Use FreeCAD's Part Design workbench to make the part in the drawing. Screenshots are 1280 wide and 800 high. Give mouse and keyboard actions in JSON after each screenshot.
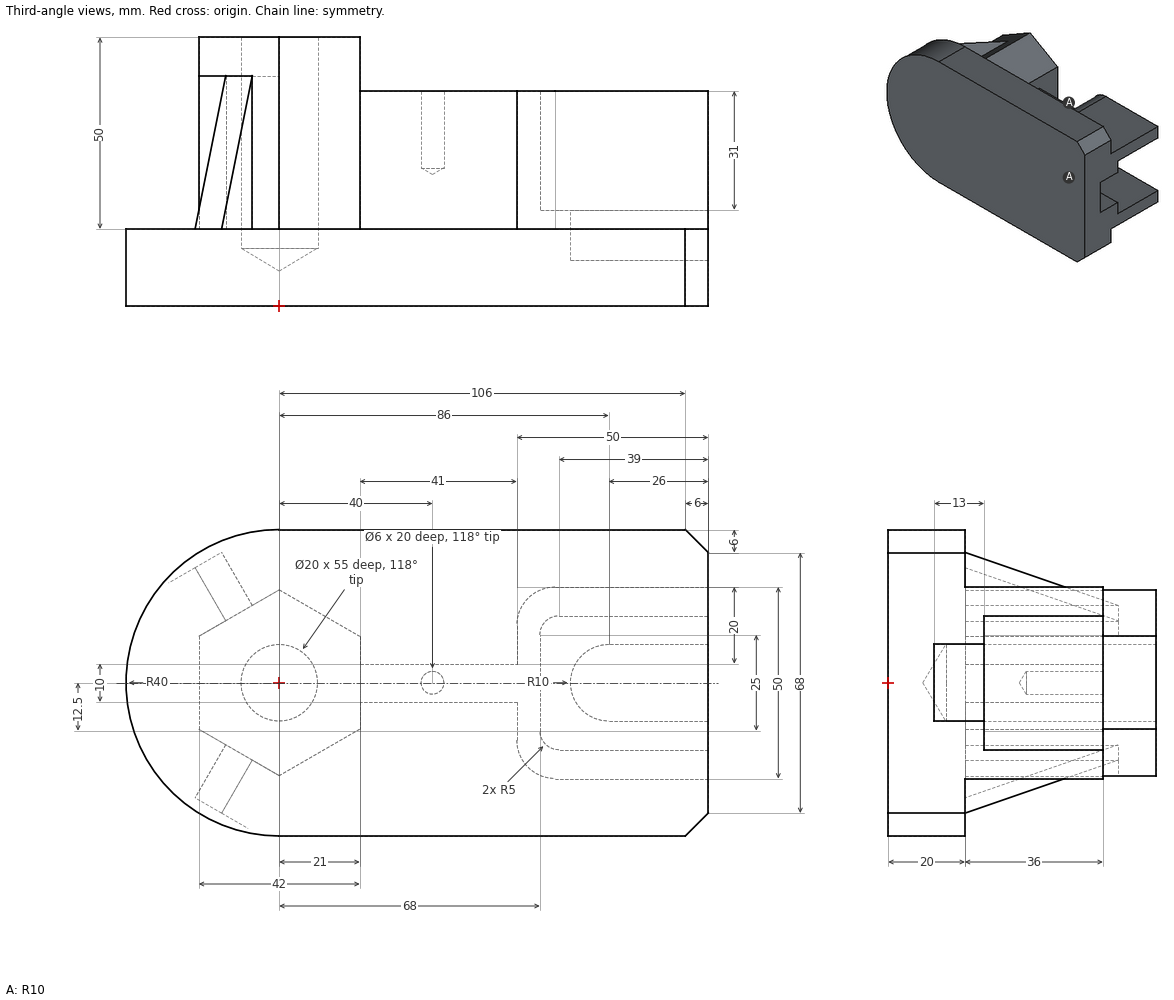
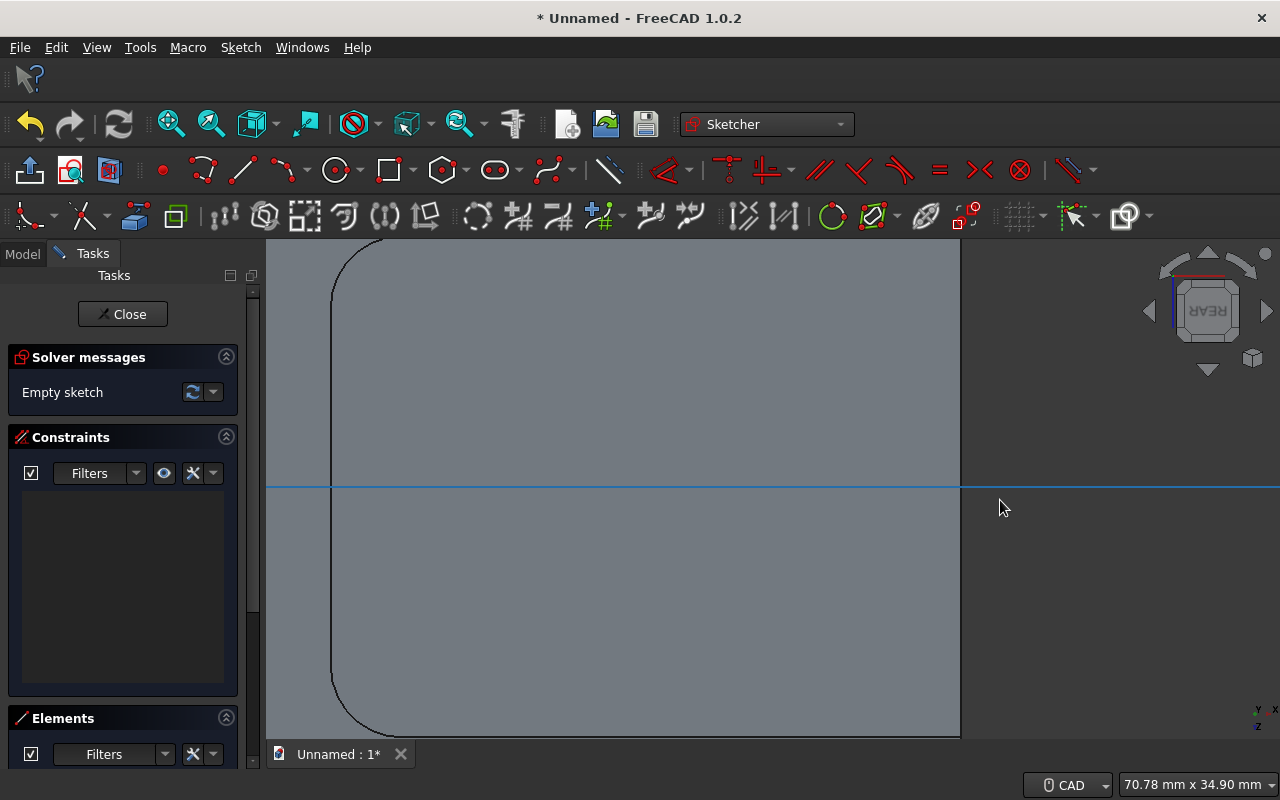
{"action": "left_click", "coordinate": [204, 170]}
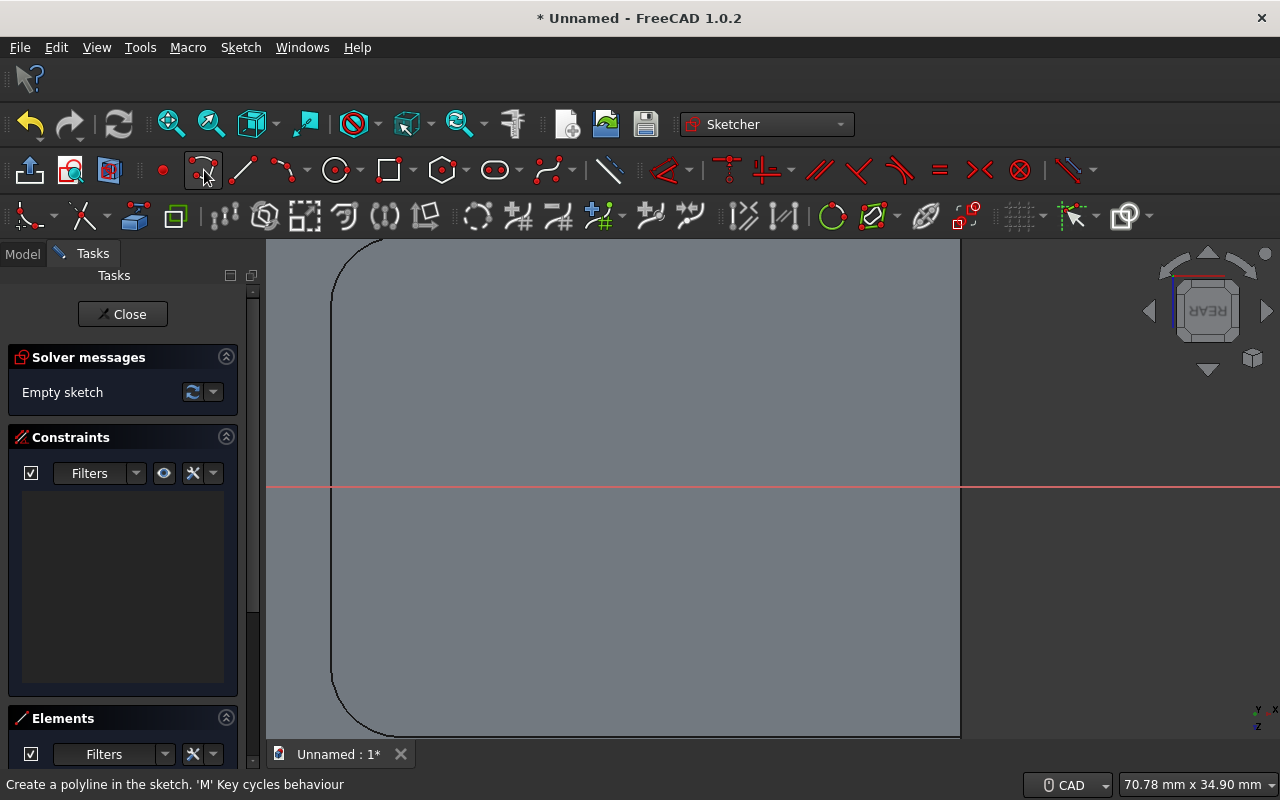
{"action": "left_click", "coordinate": [589, 630]}
{"action": "left_click", "coordinate": [961, 630]}
{"action": "left_click", "coordinate": [961, 344]}
{"action": "left_click", "coordinate": [589, 344]}
{"action": "right_click", "coordinate": [589, 344]}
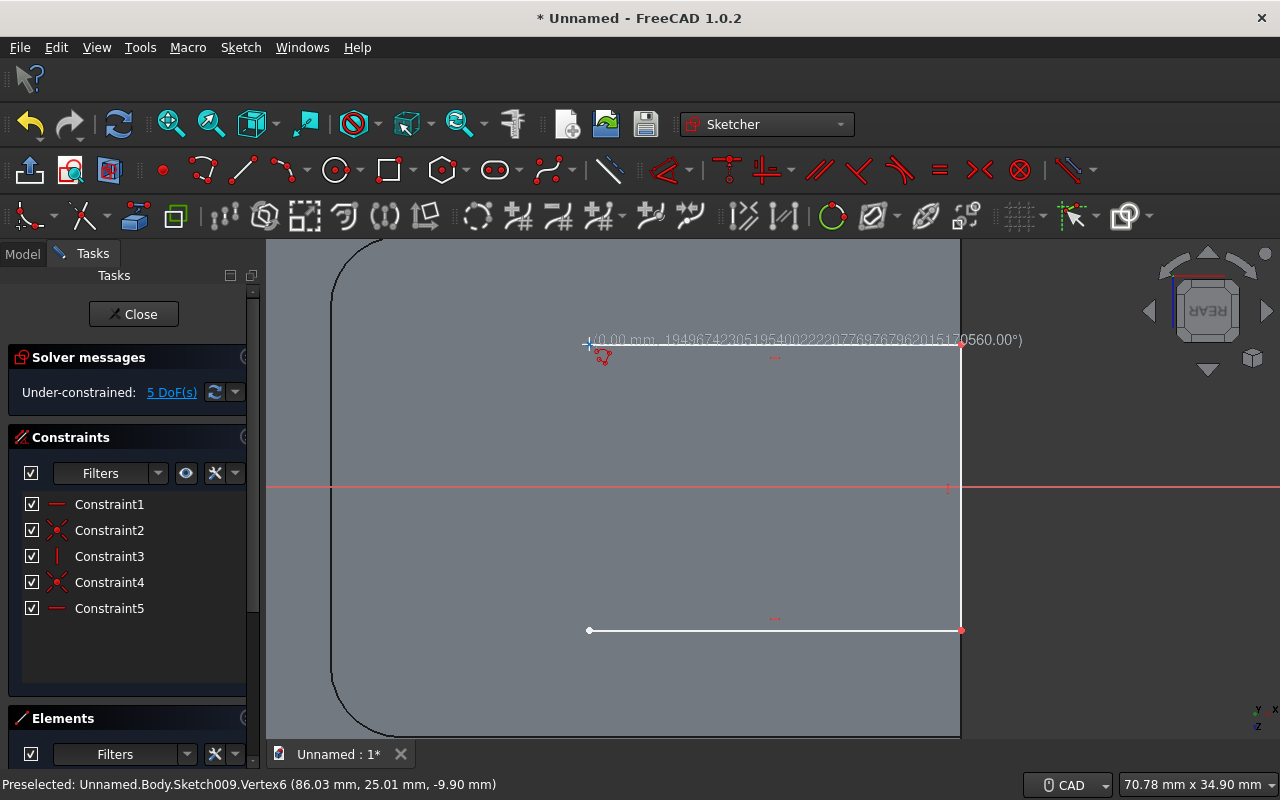
{"action": "left_click", "coordinate": [284, 170]}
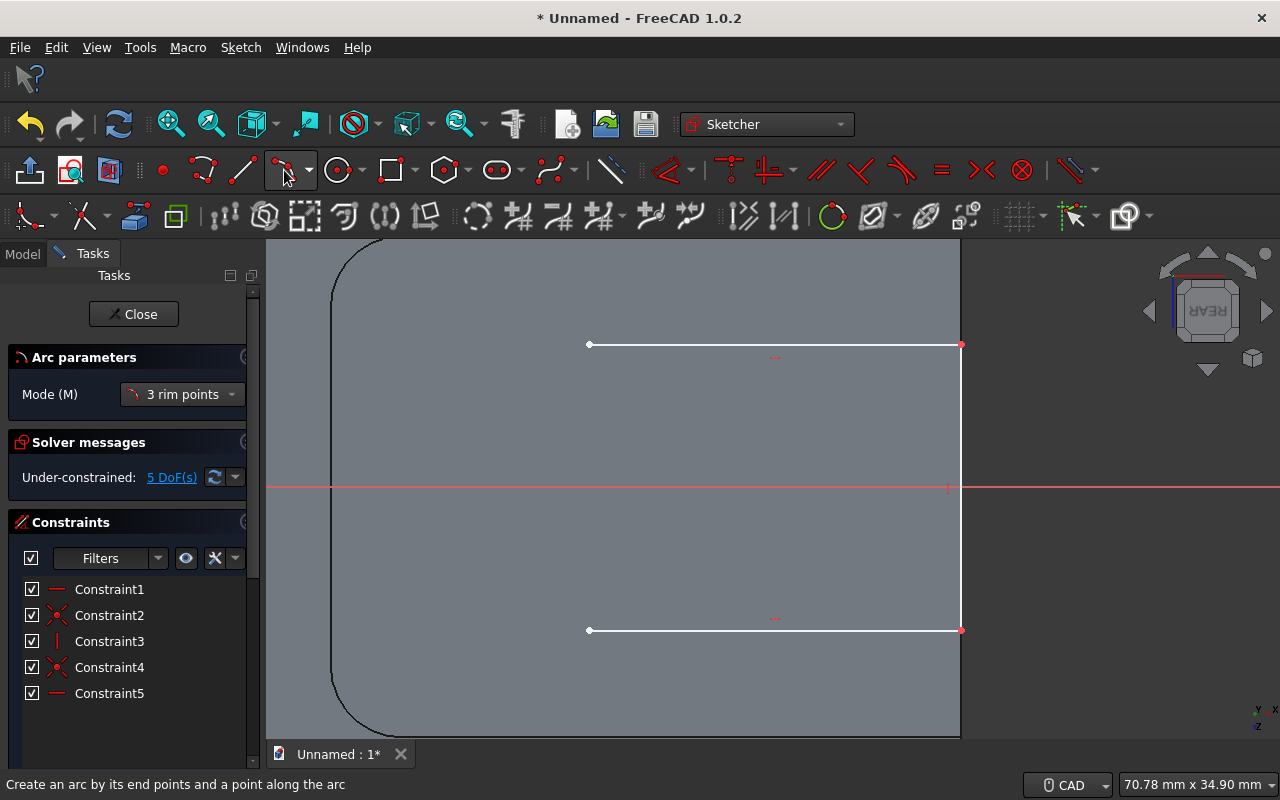
{"action": "left_click", "coordinate": [589, 345]}
{"action": "left_click", "coordinate": [589, 631]}
{"action": "left_click", "coordinate": [452, 442]}
{"action": "key", "text": "Escape"}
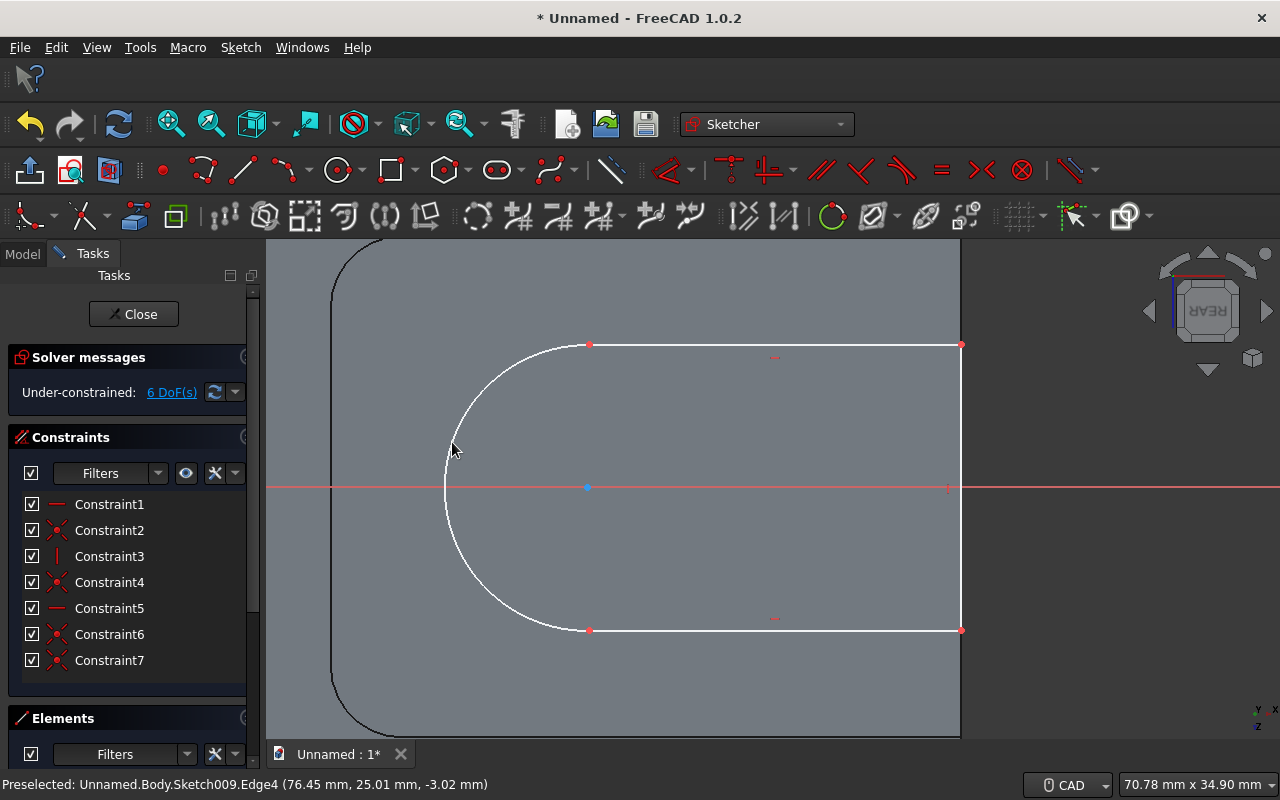
{"action": "left_click", "coordinate": [701, 631]}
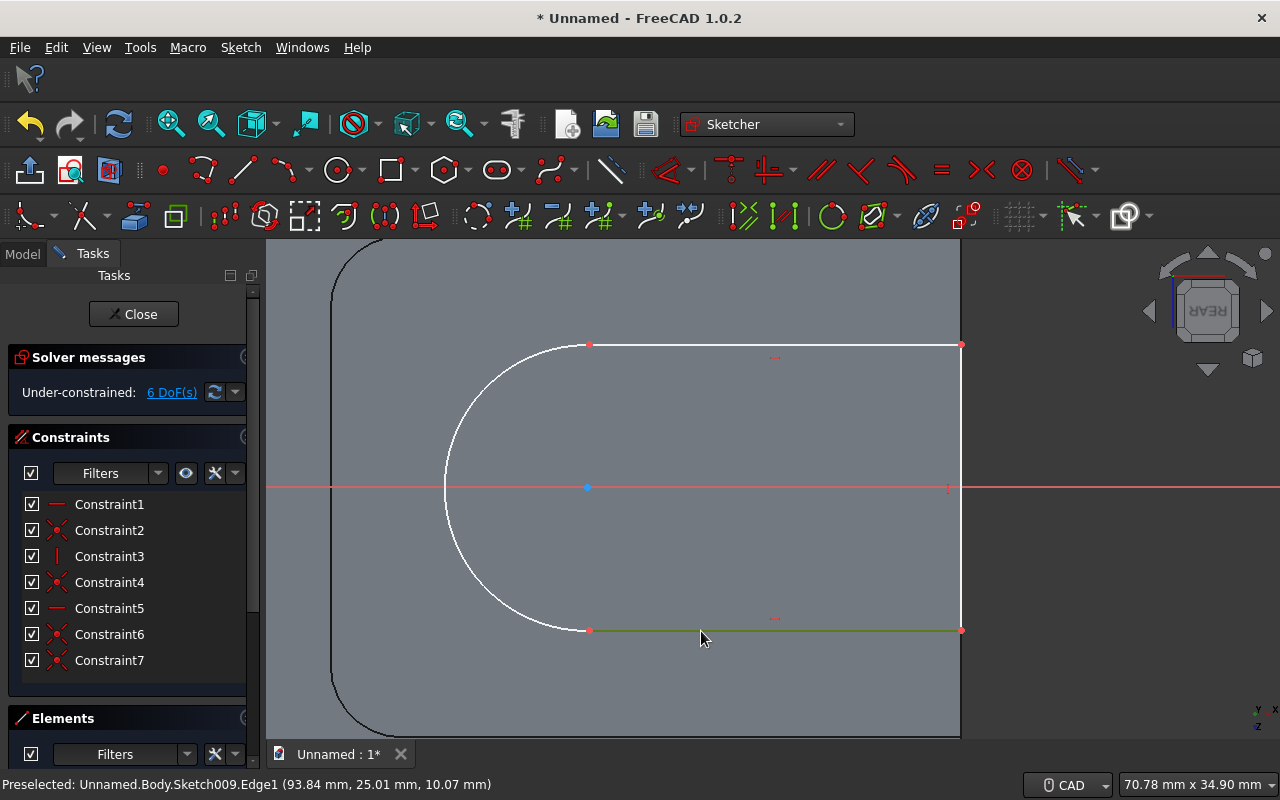
{"action": "left_click", "coordinate": [472, 404]}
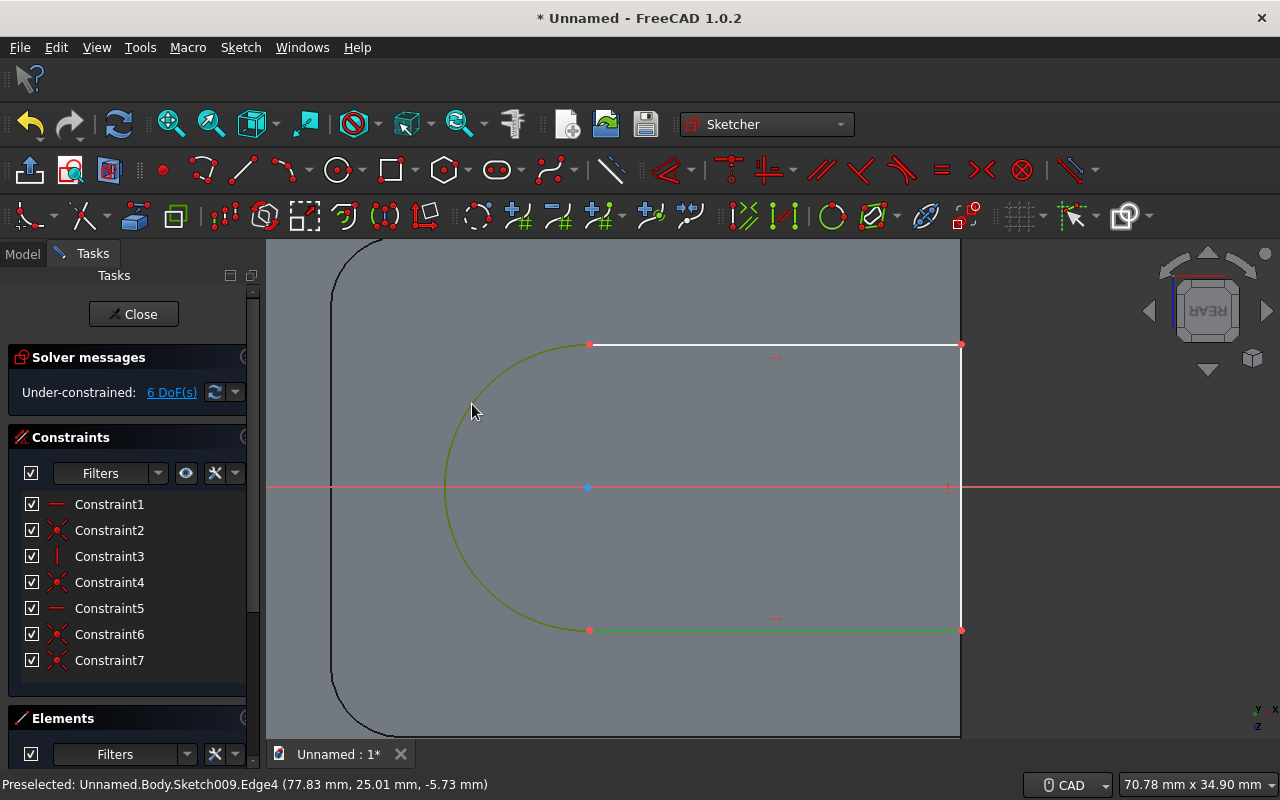
{"action": "left_click", "coordinate": [902, 170]}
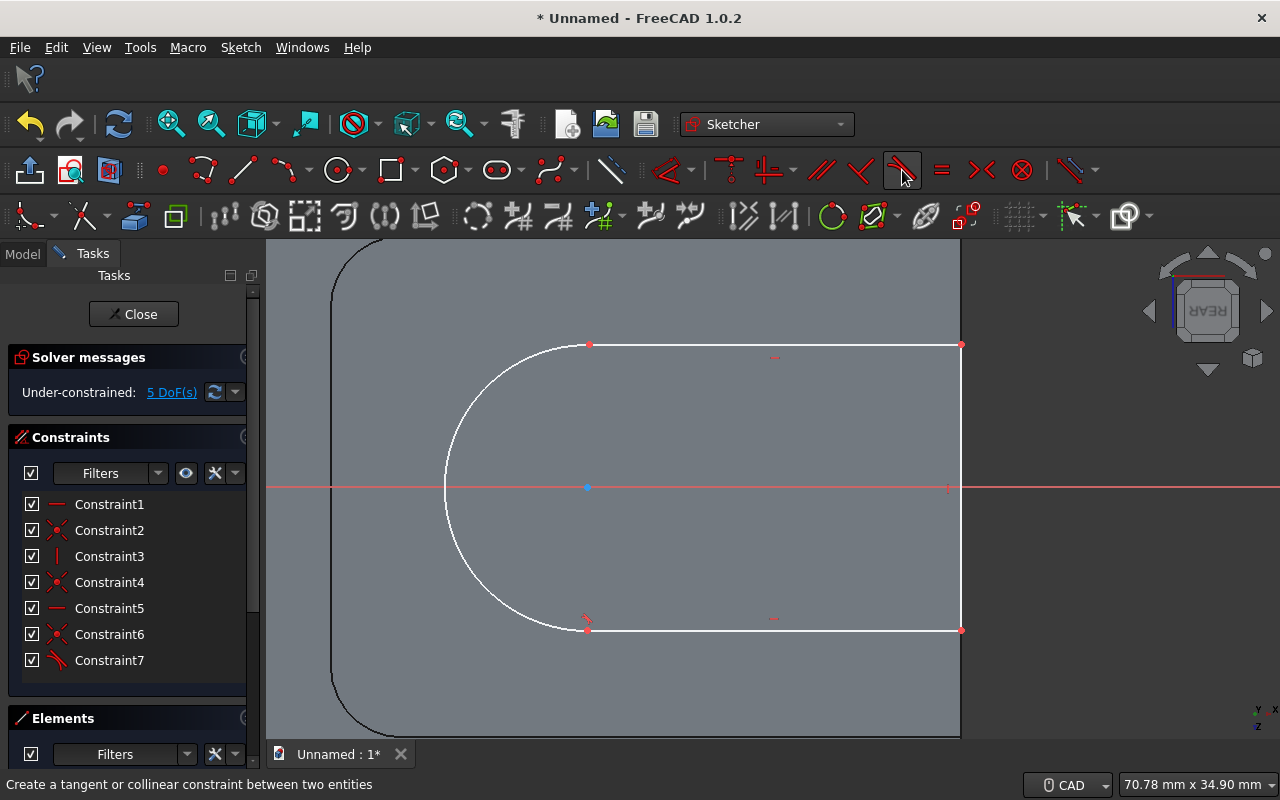
{"action": "left_click", "coordinate": [849, 345]}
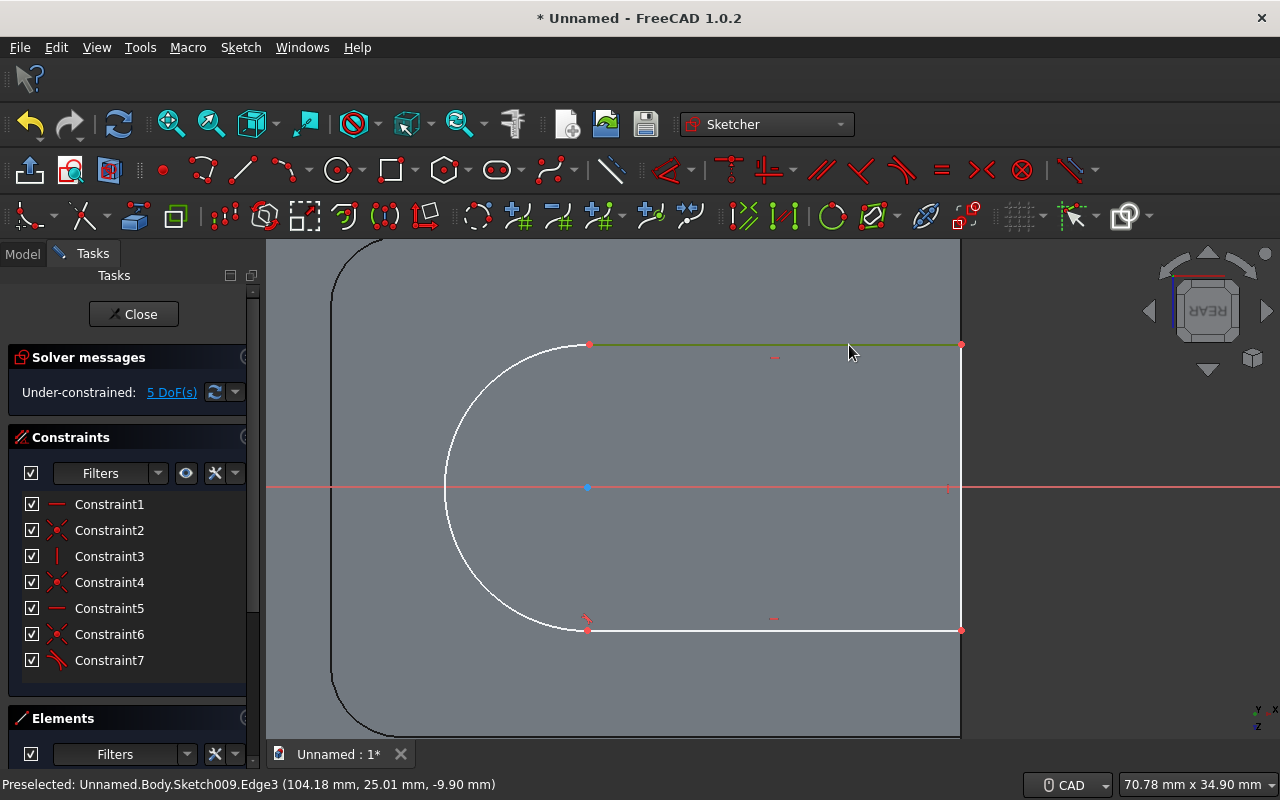
{"action": "left_click", "coordinate": [473, 403]}